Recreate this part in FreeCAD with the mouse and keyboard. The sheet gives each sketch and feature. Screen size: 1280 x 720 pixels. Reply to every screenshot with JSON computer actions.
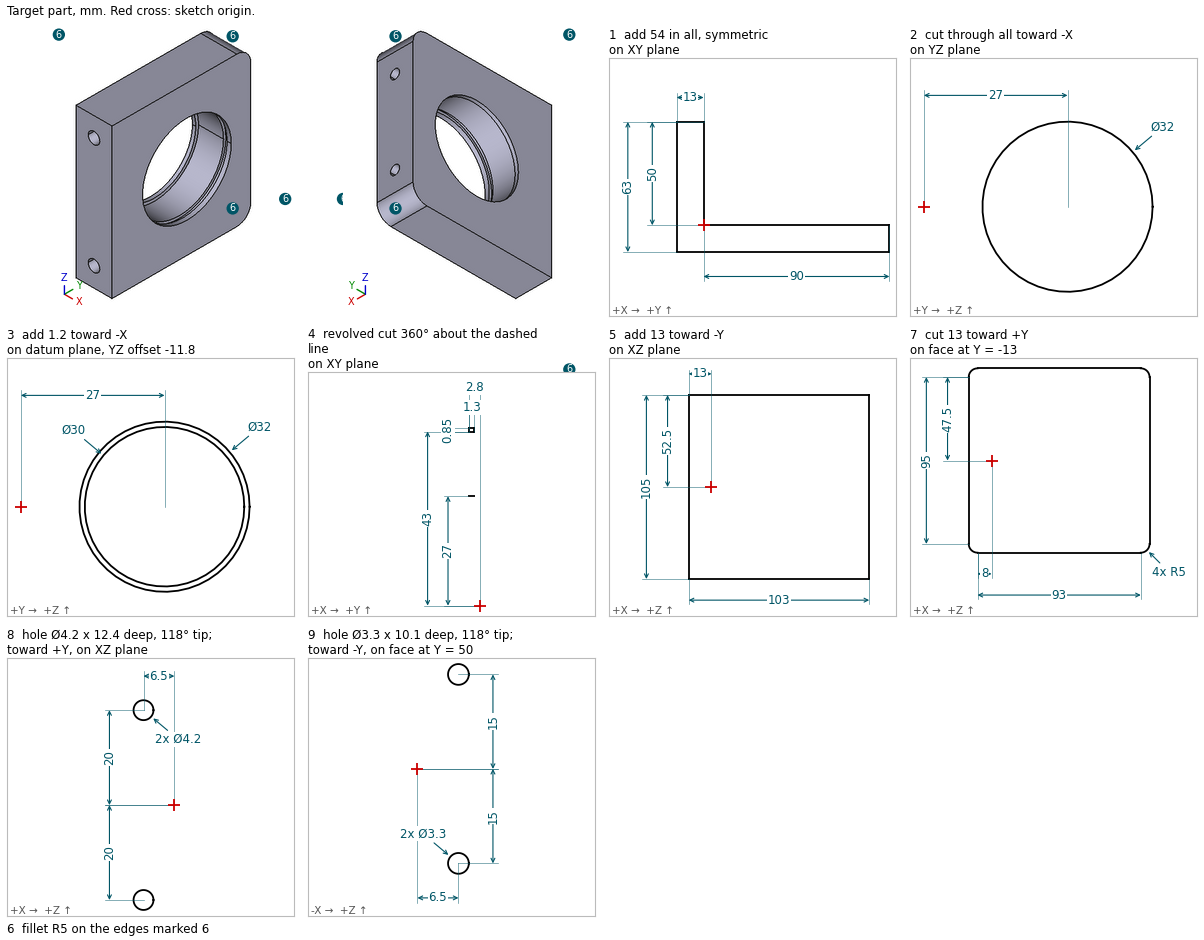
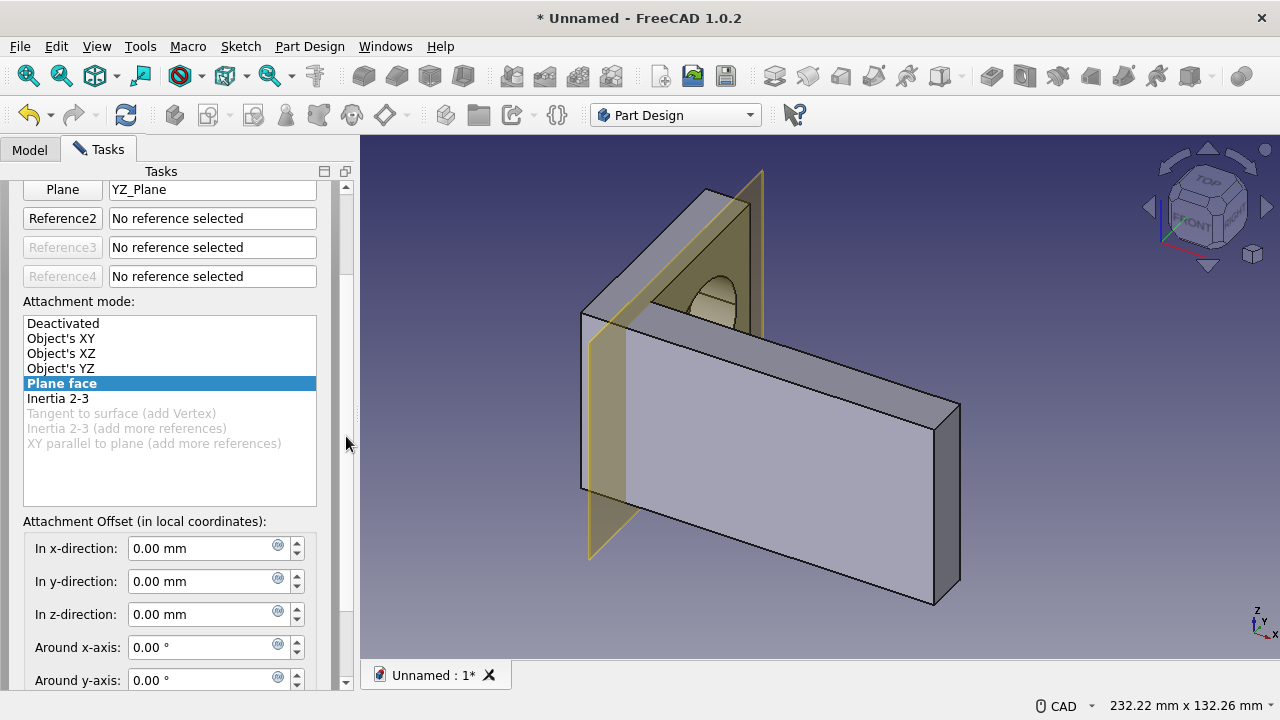
{"action": "triple_click", "coordinate": [210, 614]}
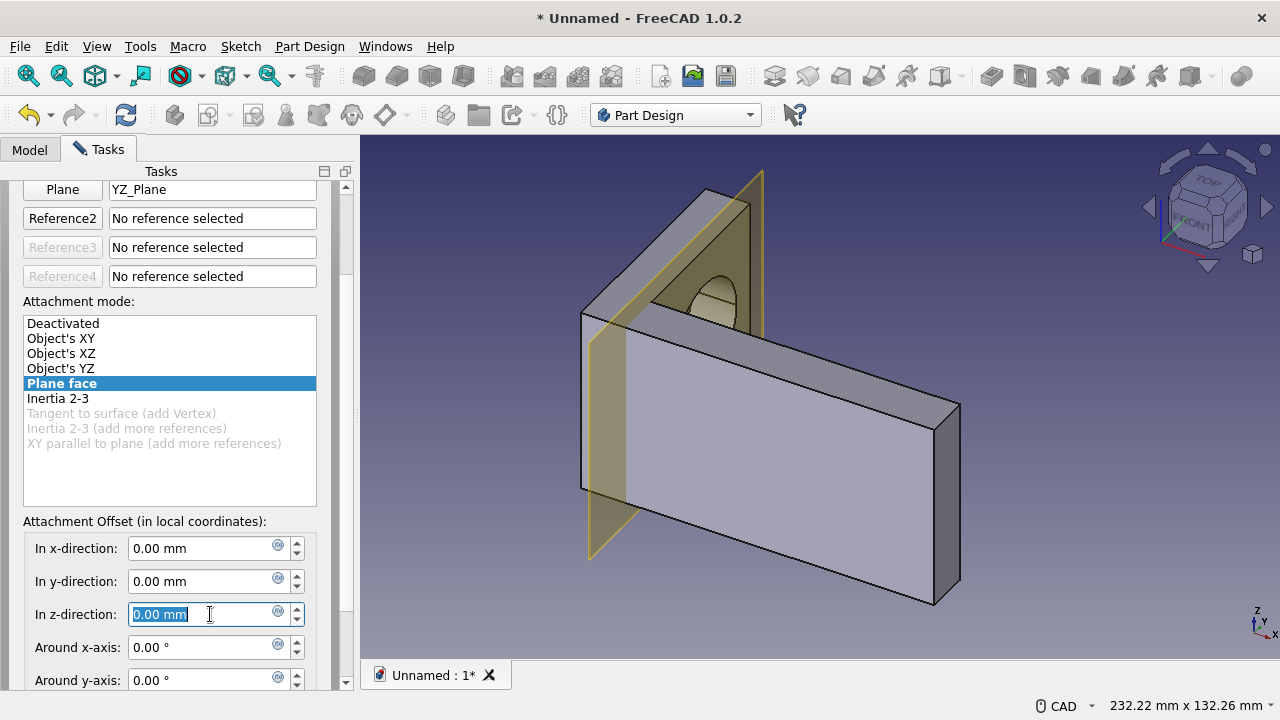
{"action": "type", "text": "-11.8"}
{"action": "key", "text": "Tab"}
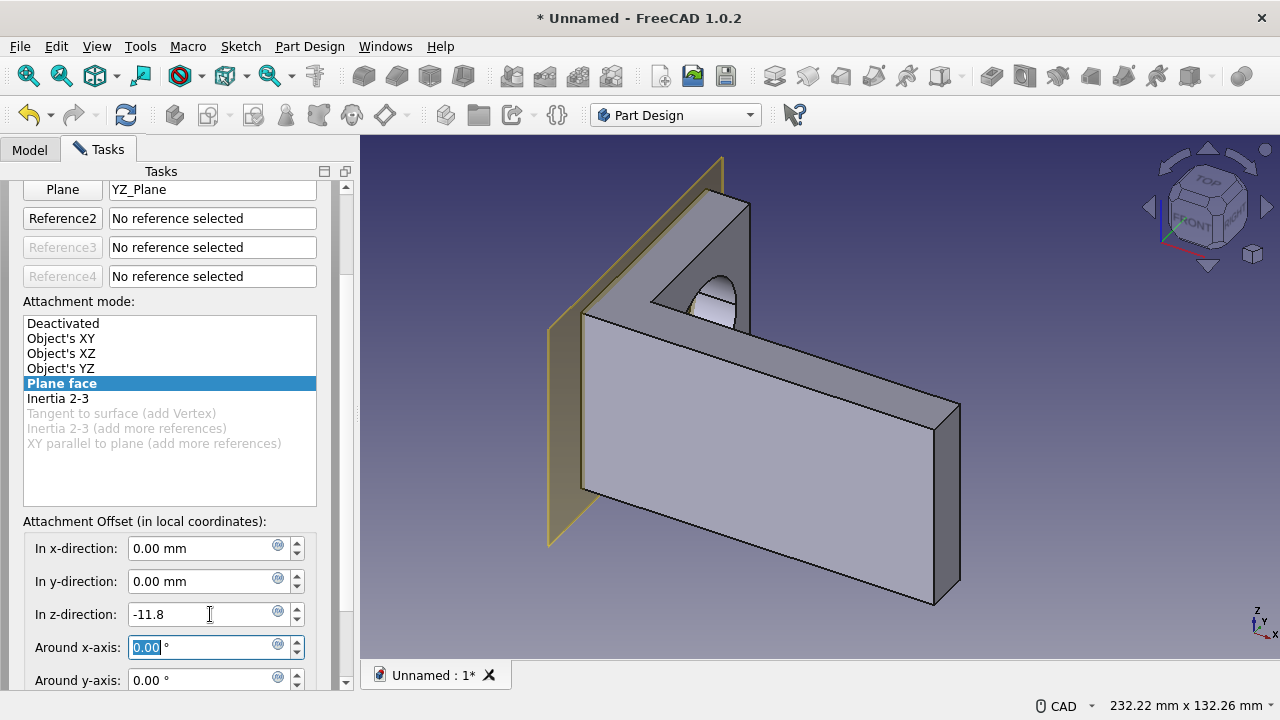
{"action": "scroll", "coordinate": [346, 436], "scroll_direction": "up", "scroll_amount": 3}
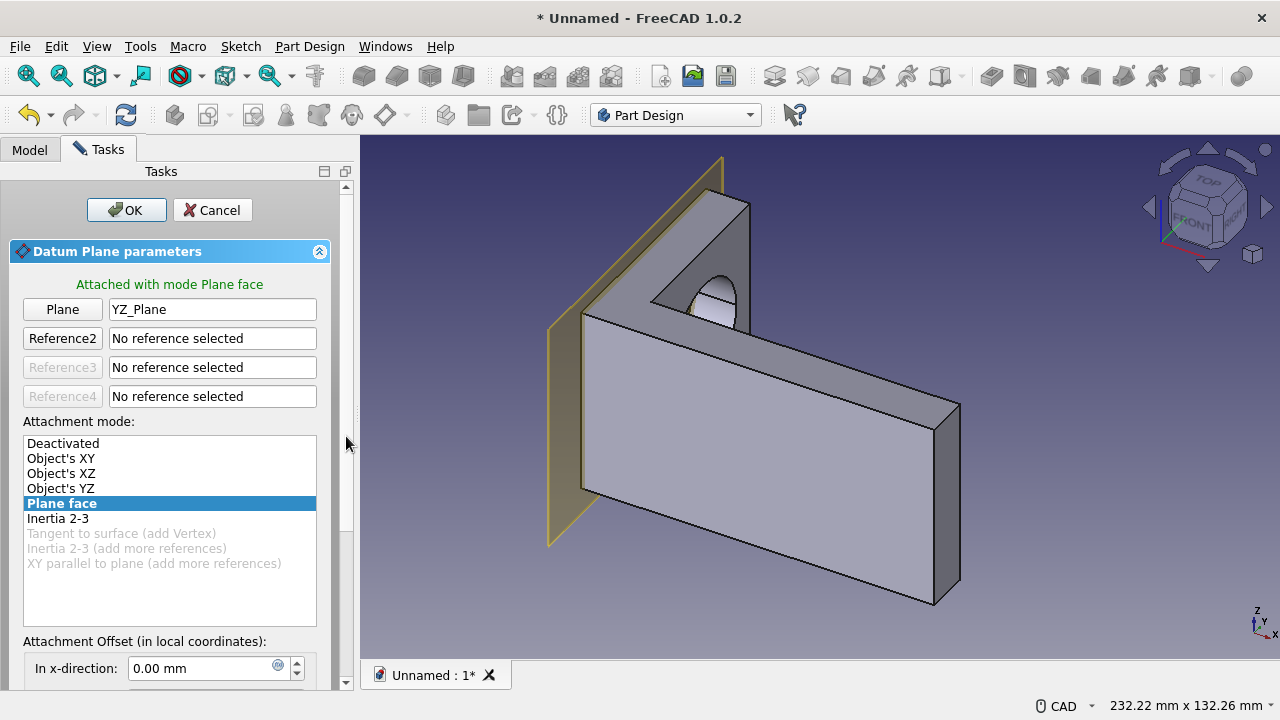
{"action": "left_click", "coordinate": [127, 210]}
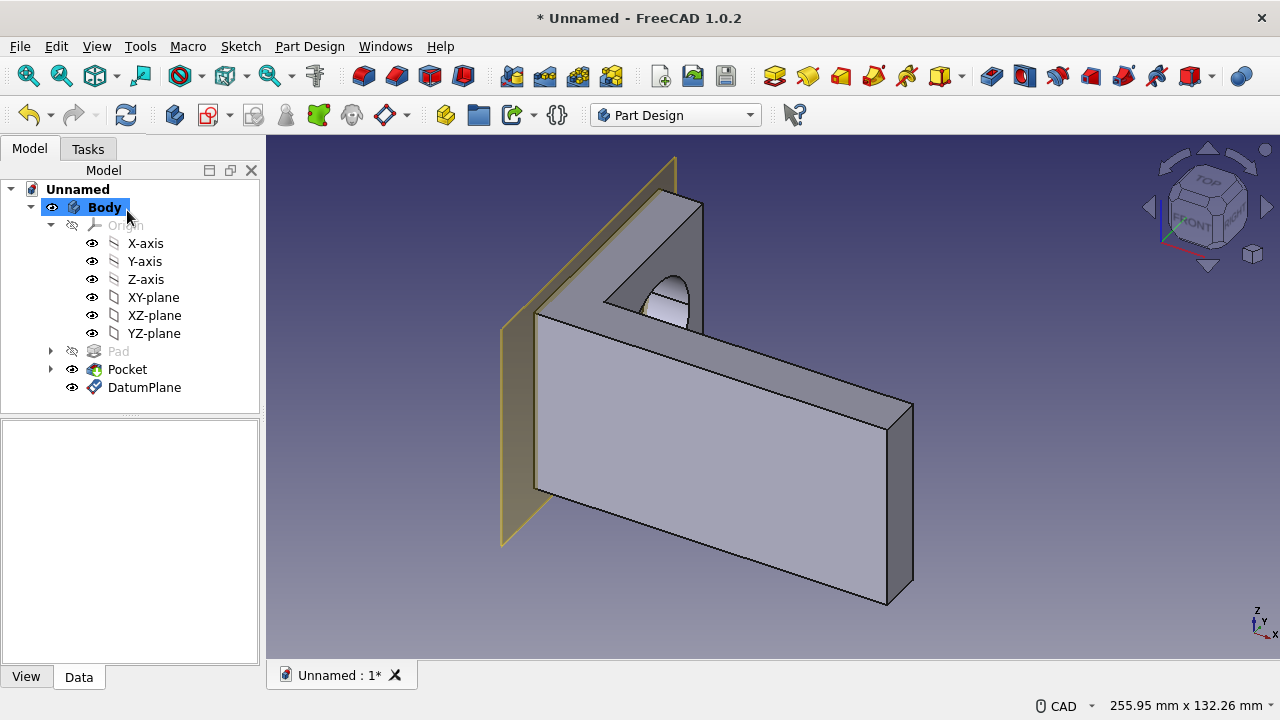
{"action": "left_click", "coordinate": [117, 387]}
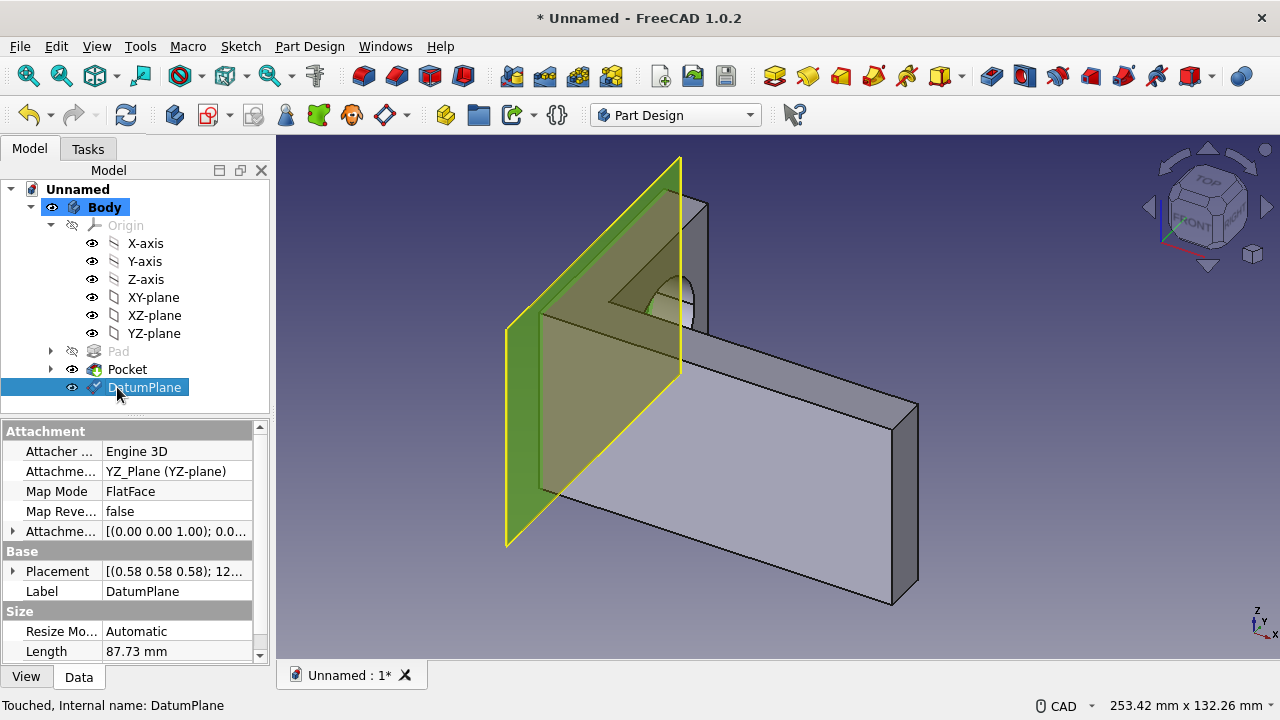
{"action": "left_click", "coordinate": [208, 116]}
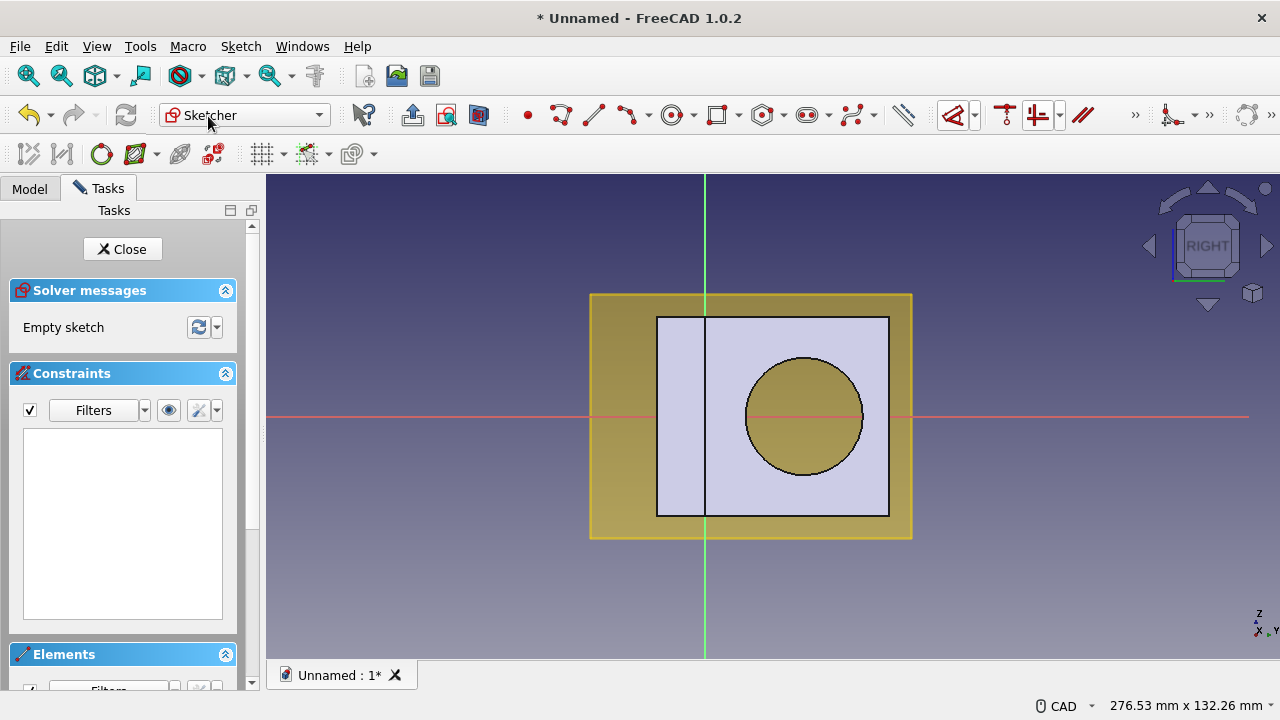
{"action": "left_click", "coordinate": [479, 116]}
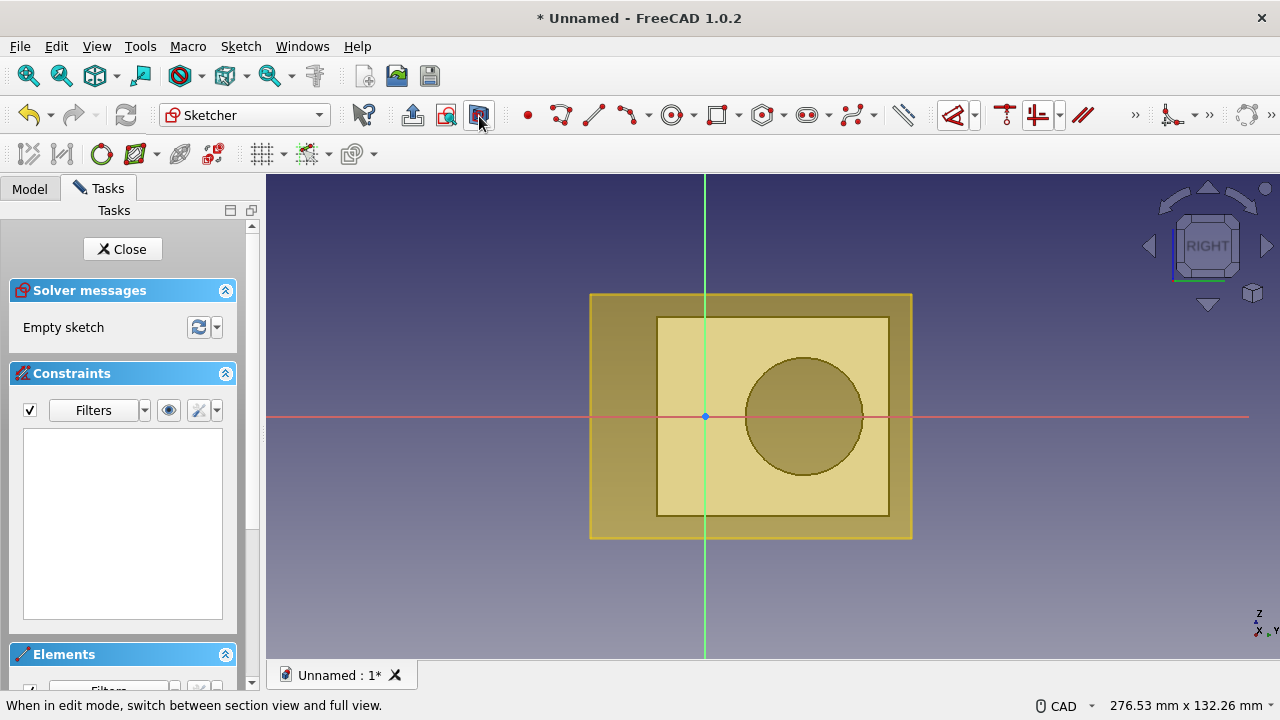
{"action": "scroll", "coordinate": [830, 416], "scroll_direction": "up", "scroll_amount": 5}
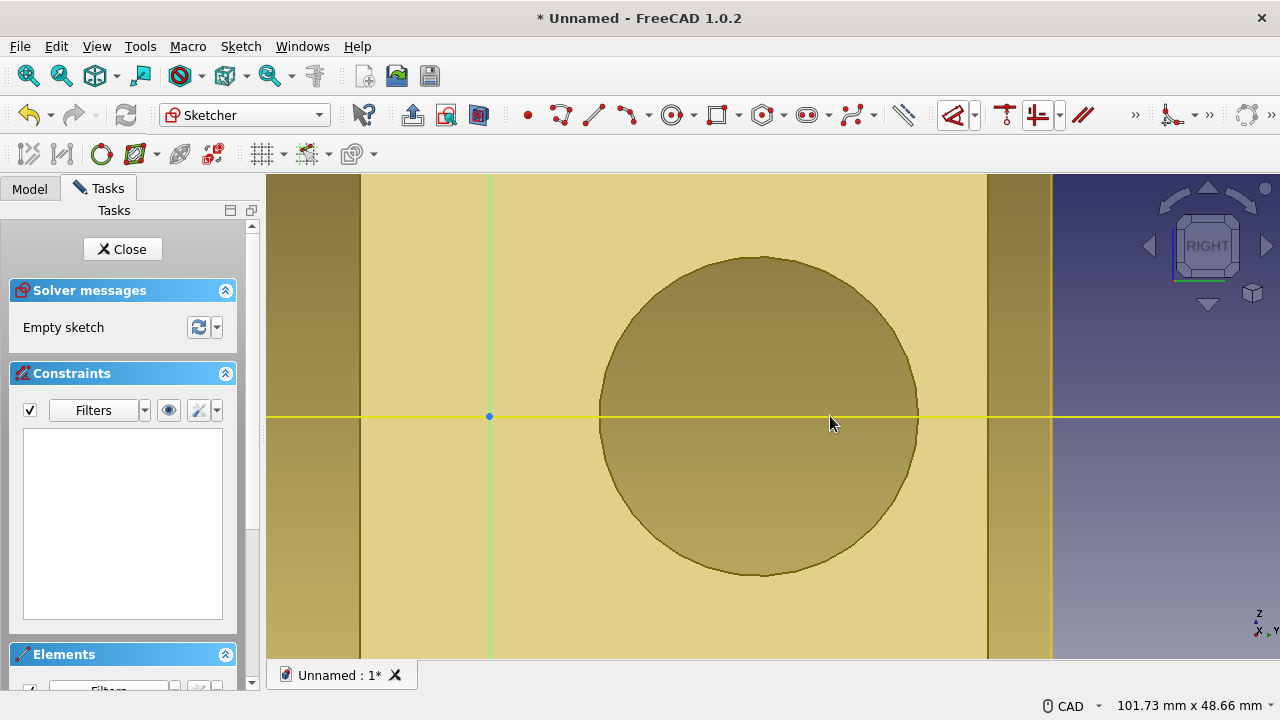
{"action": "left_click", "coordinate": [672, 116]}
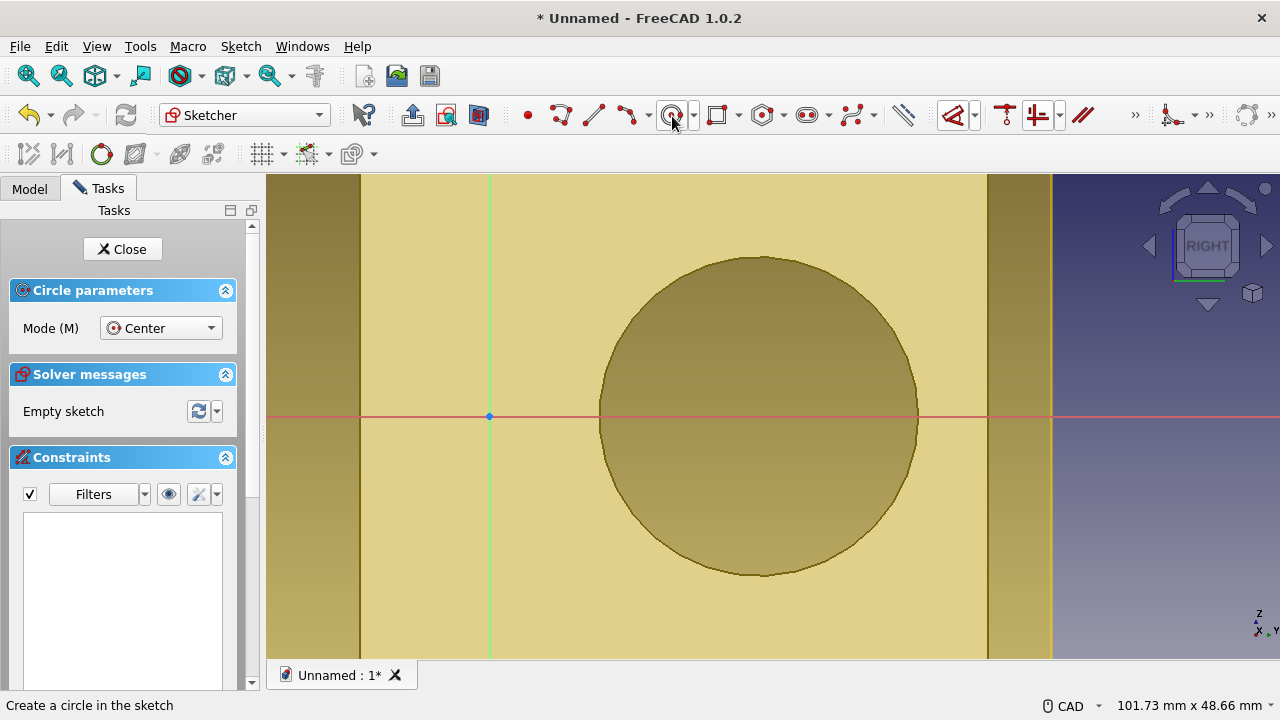
{"action": "left_click", "coordinate": [759, 416]}
{"action": "left_click", "coordinate": [872, 304]}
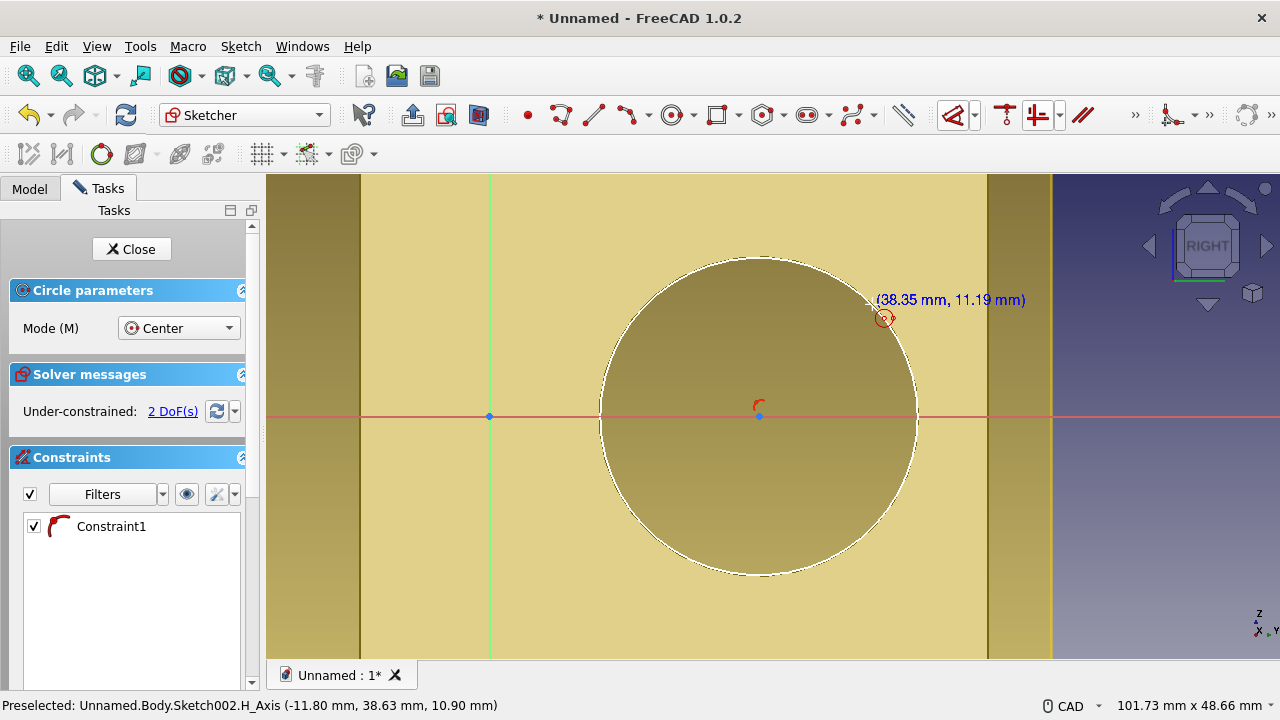
{"action": "left_click", "coordinate": [759, 416]}